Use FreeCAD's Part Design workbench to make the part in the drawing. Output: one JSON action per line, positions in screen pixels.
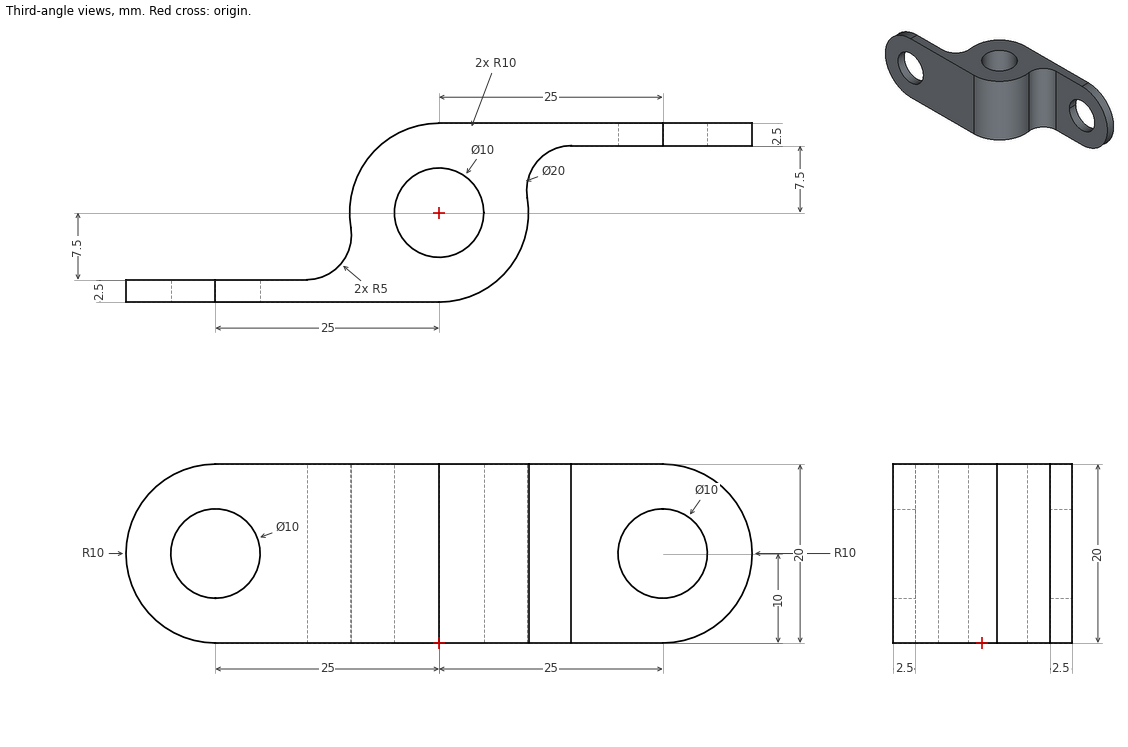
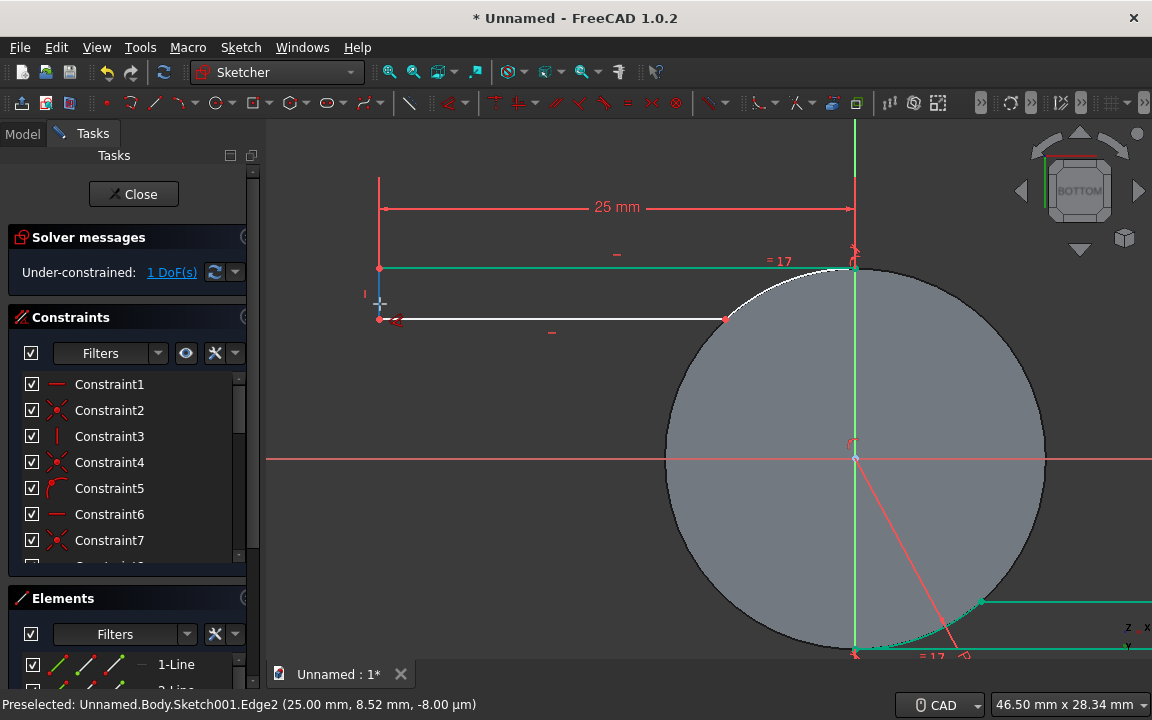
{"action": "left_click", "coordinate": [379, 304]}
{"action": "left_click", "coordinate": [345, 294]}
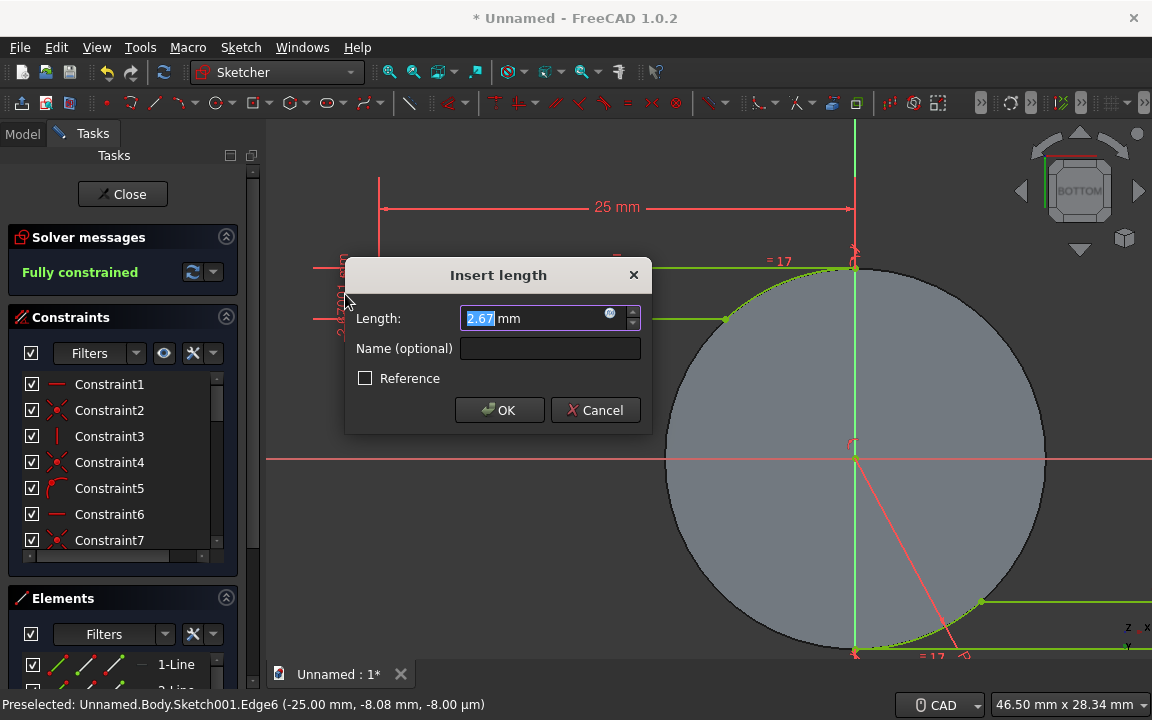
{"action": "type", "text": "2.5"}
{"action": "key", "text": "Return"}
{"action": "key", "text": "Escape"}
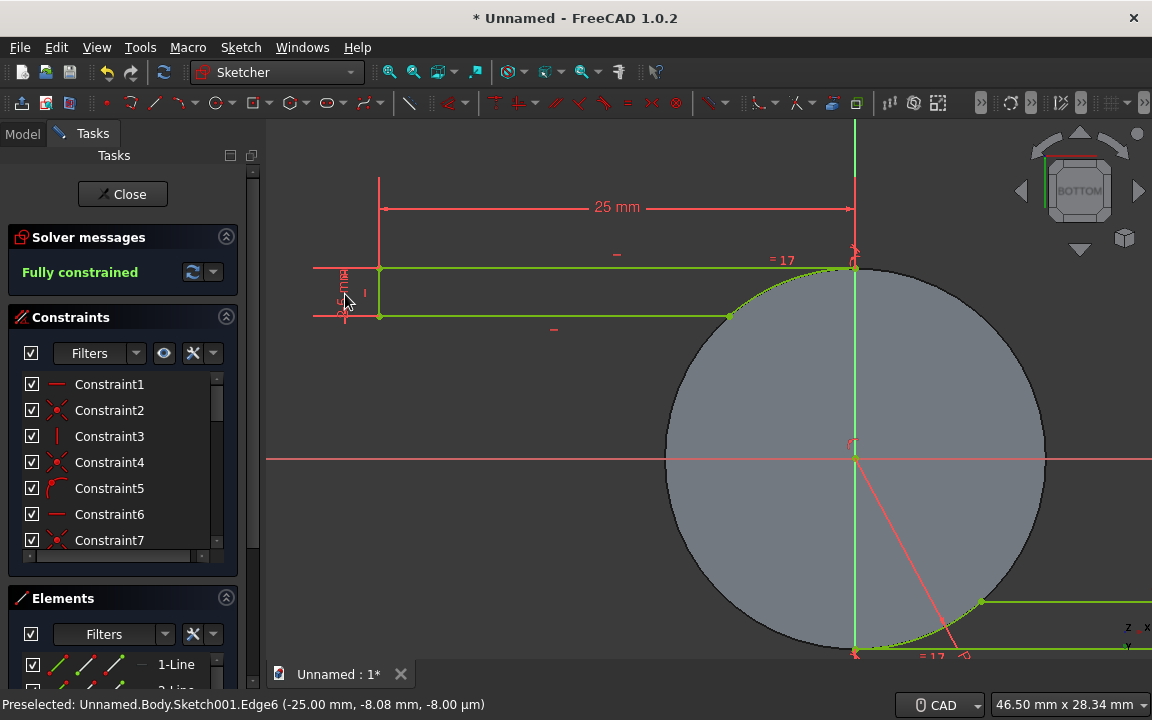
{"action": "left_click", "coordinate": [123, 194]}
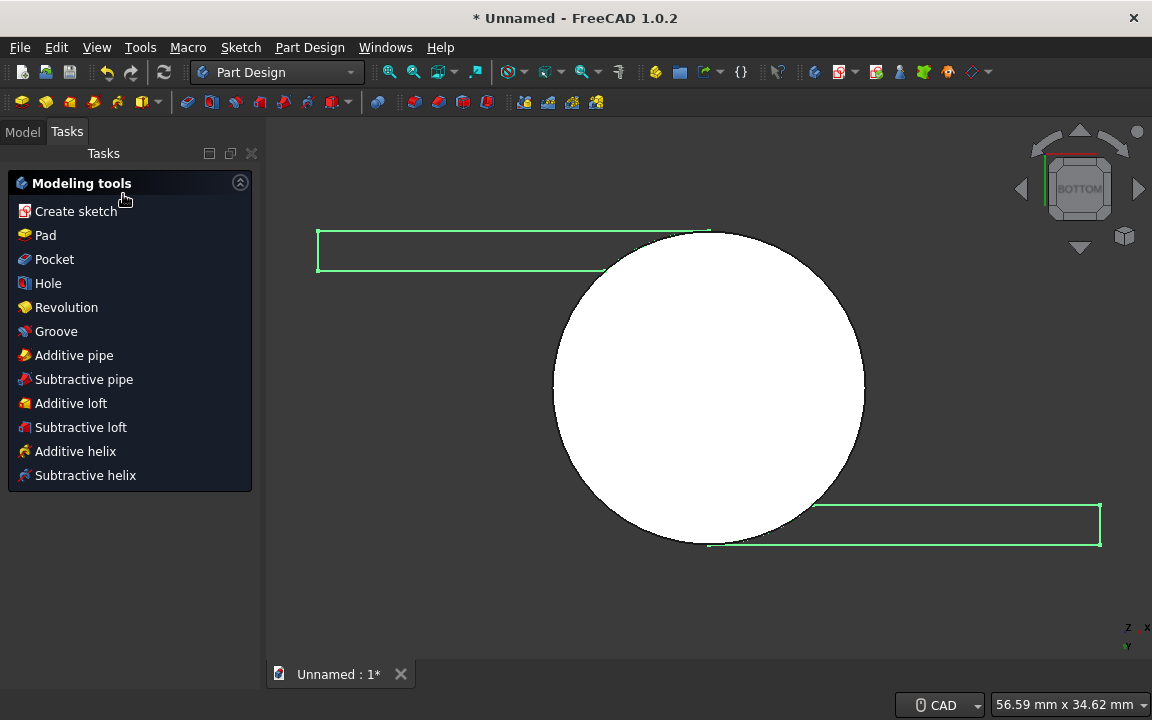
{"action": "left_click", "coordinate": [22, 102]}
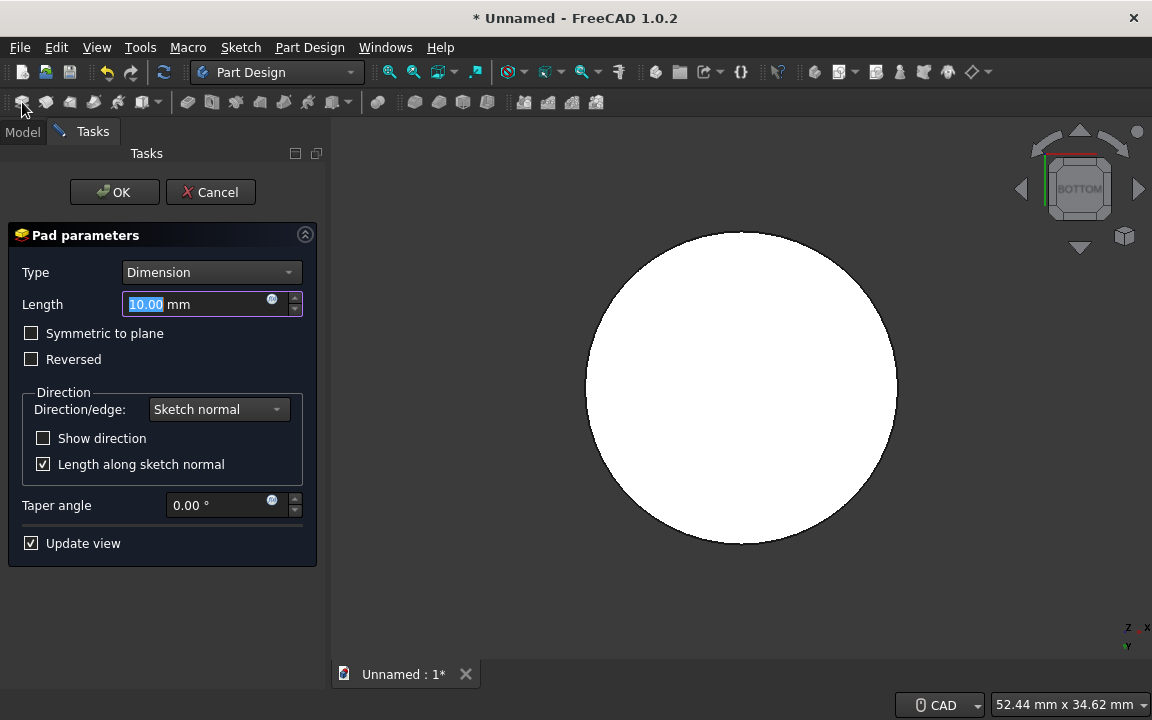
{"action": "type", "text": "20"}
{"action": "key", "text": "Tab"}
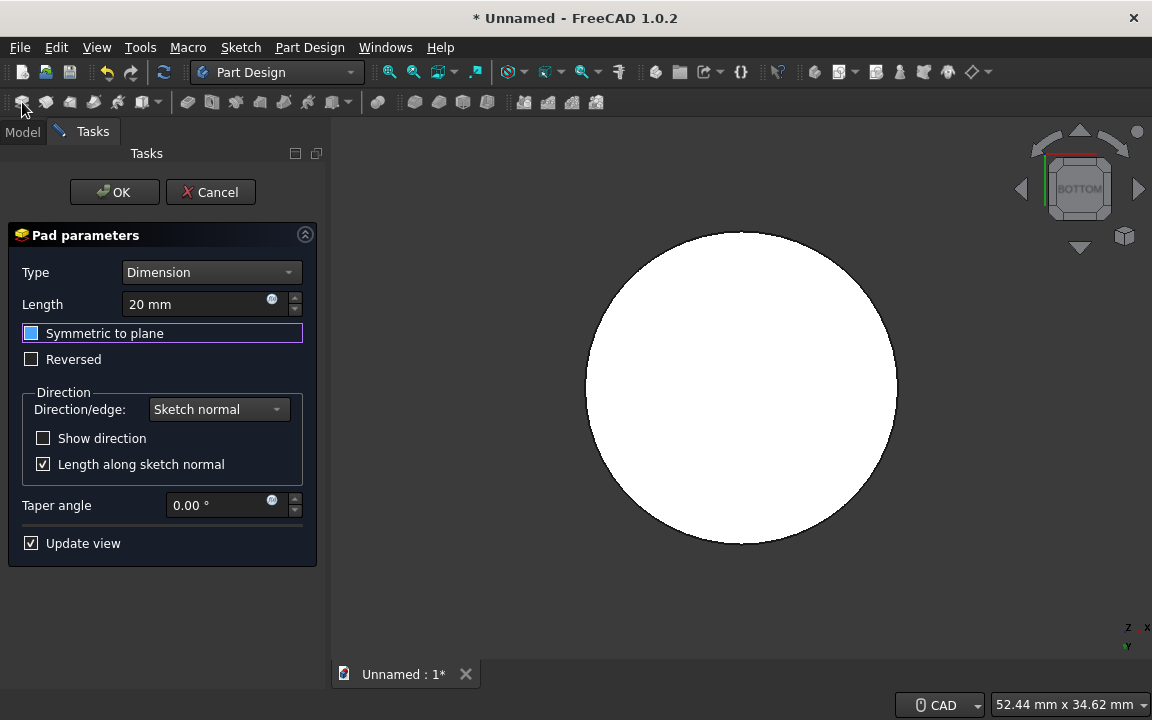
{"action": "left_click", "coordinate": [30, 359]}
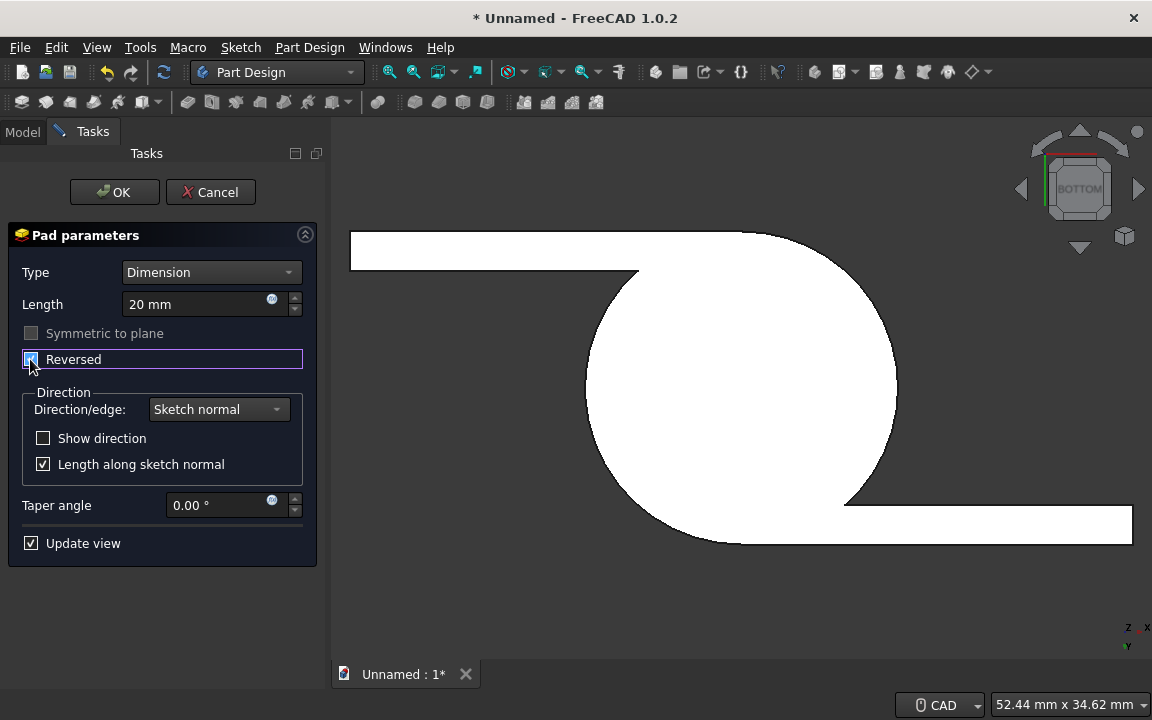
{"action": "left_click", "coordinate": [115, 192]}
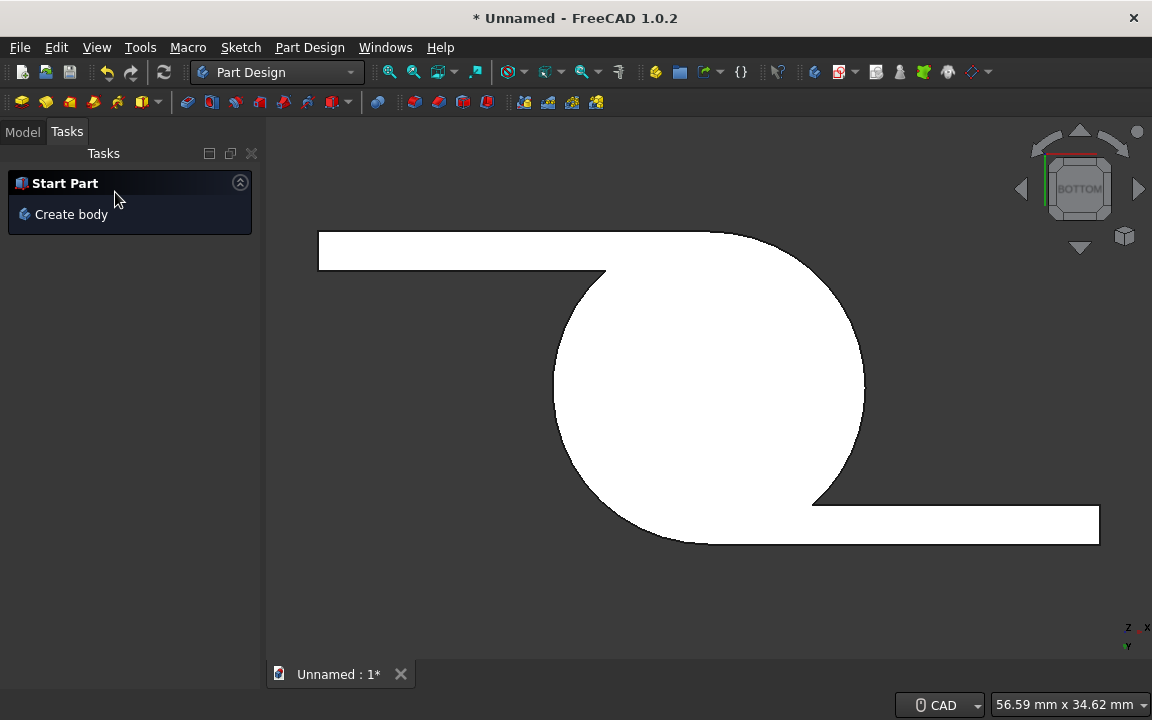
{"action": "left_click", "coordinate": [709, 387]}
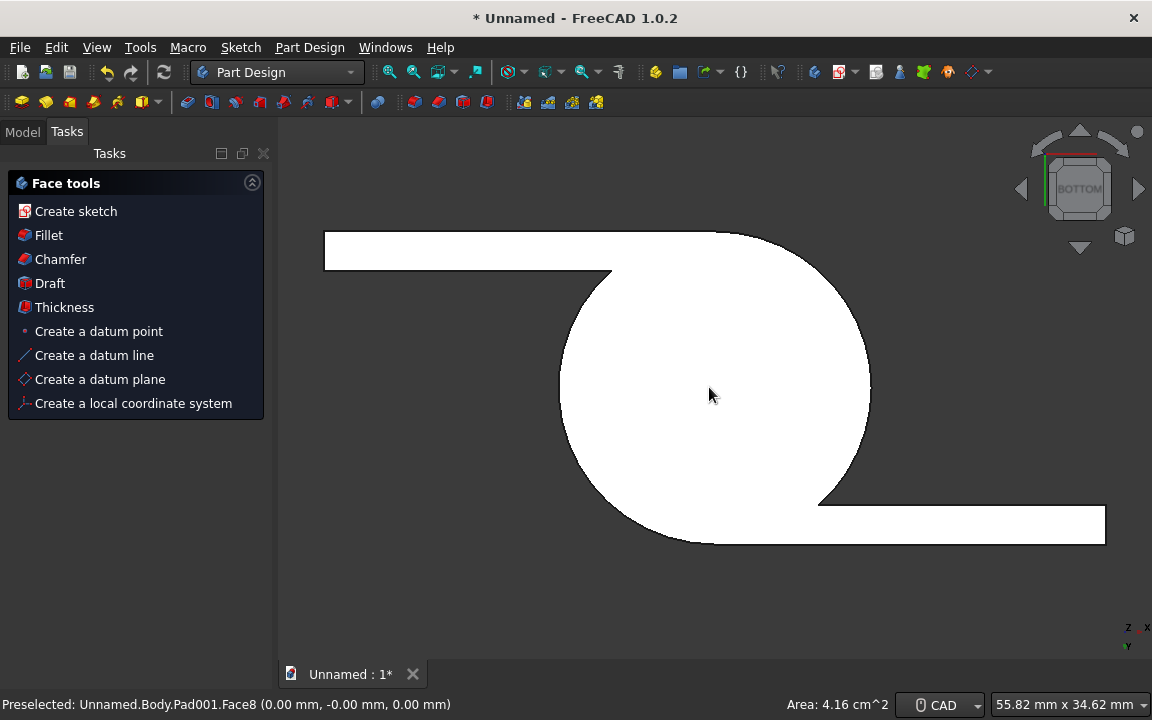
{"action": "left_click", "coordinate": [840, 72]}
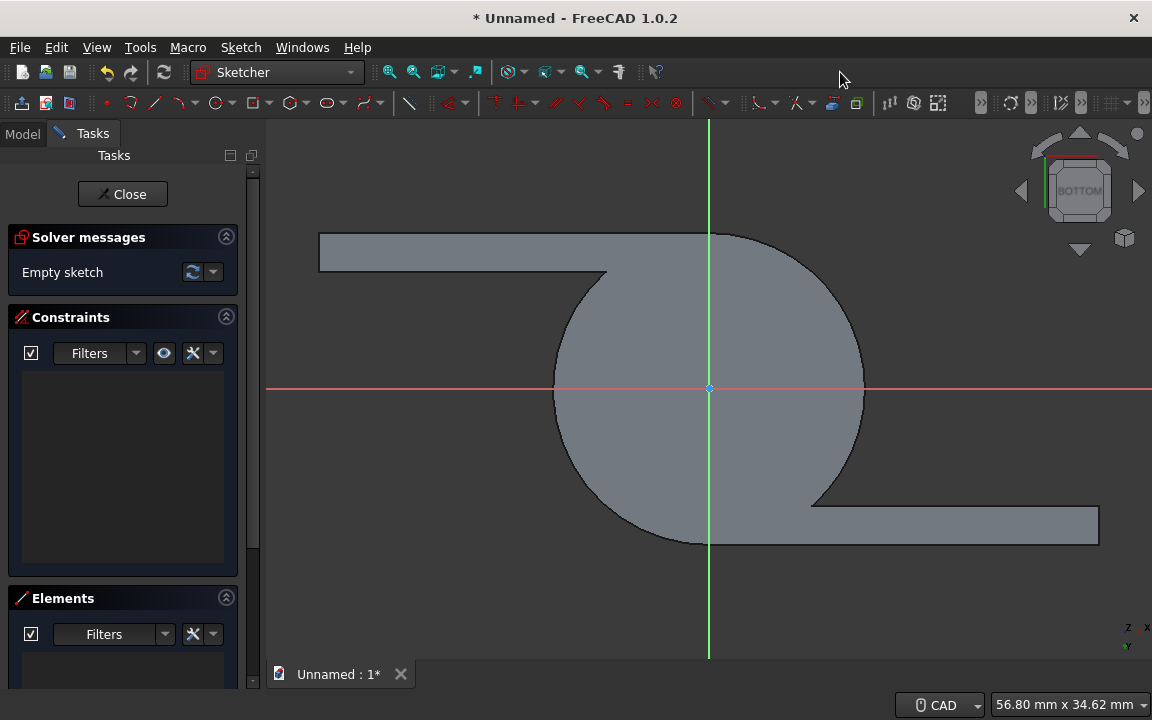
{"action": "left_click", "coordinate": [156, 104]}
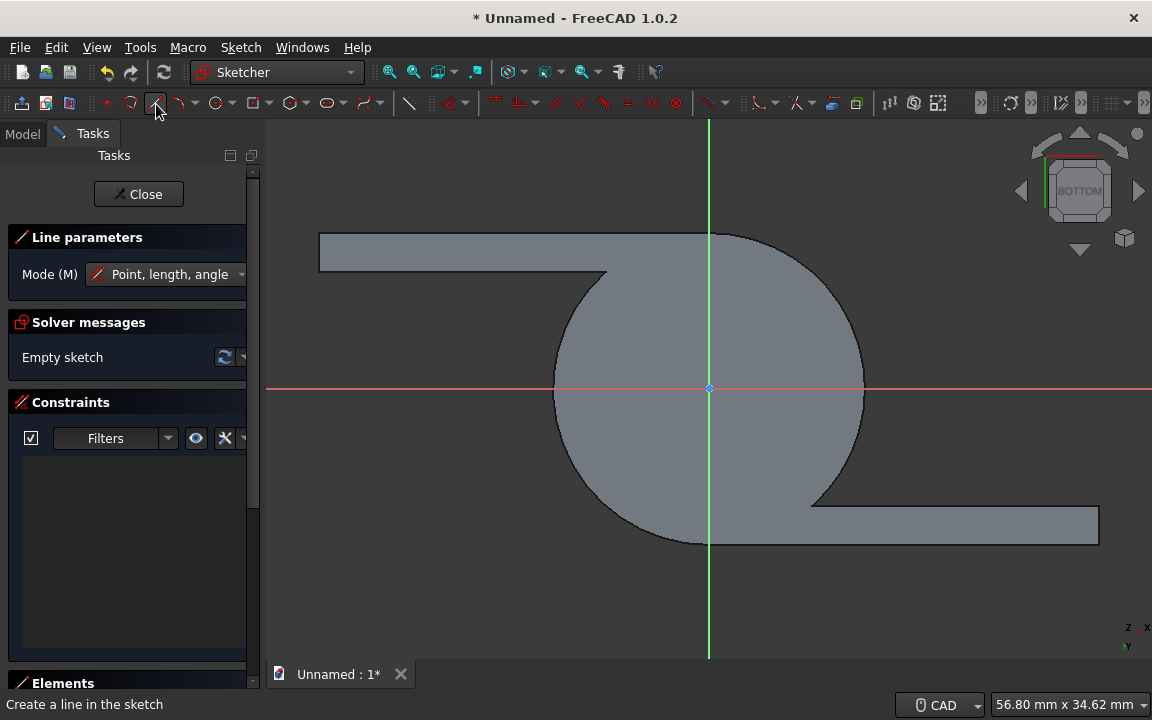
{"action": "left_click", "coordinate": [478, 272]}
{"action": "left_click", "coordinate": [606, 272]}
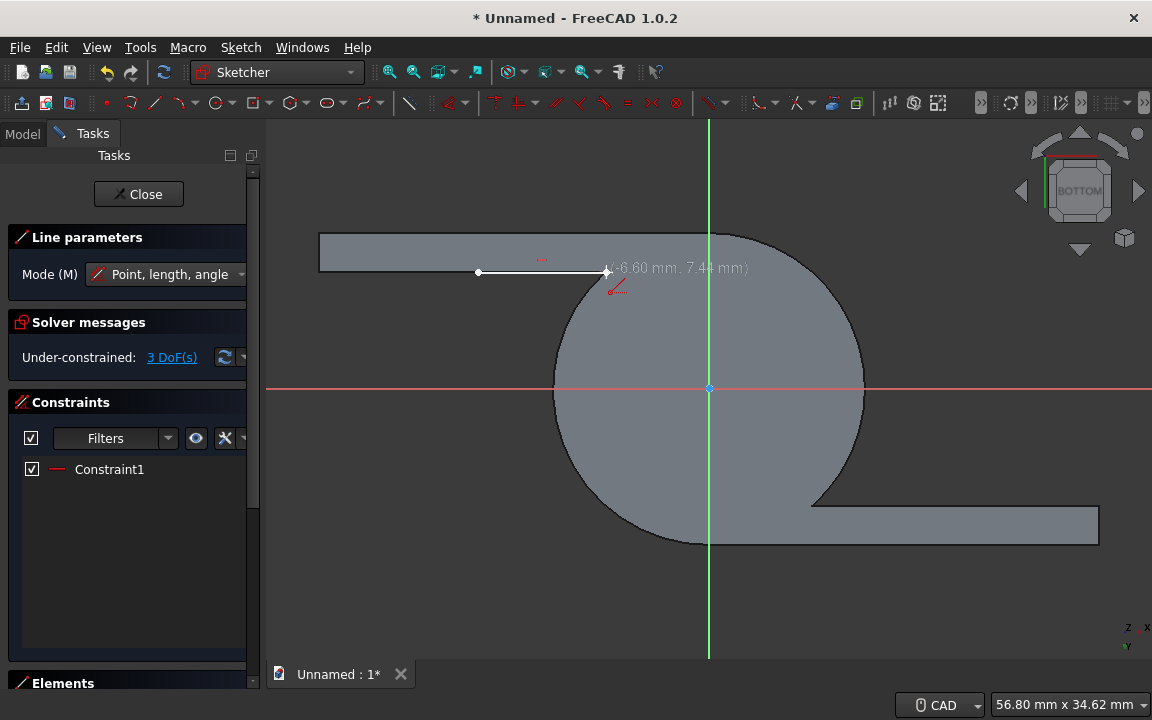
{"action": "key", "text": "g 3 a"}